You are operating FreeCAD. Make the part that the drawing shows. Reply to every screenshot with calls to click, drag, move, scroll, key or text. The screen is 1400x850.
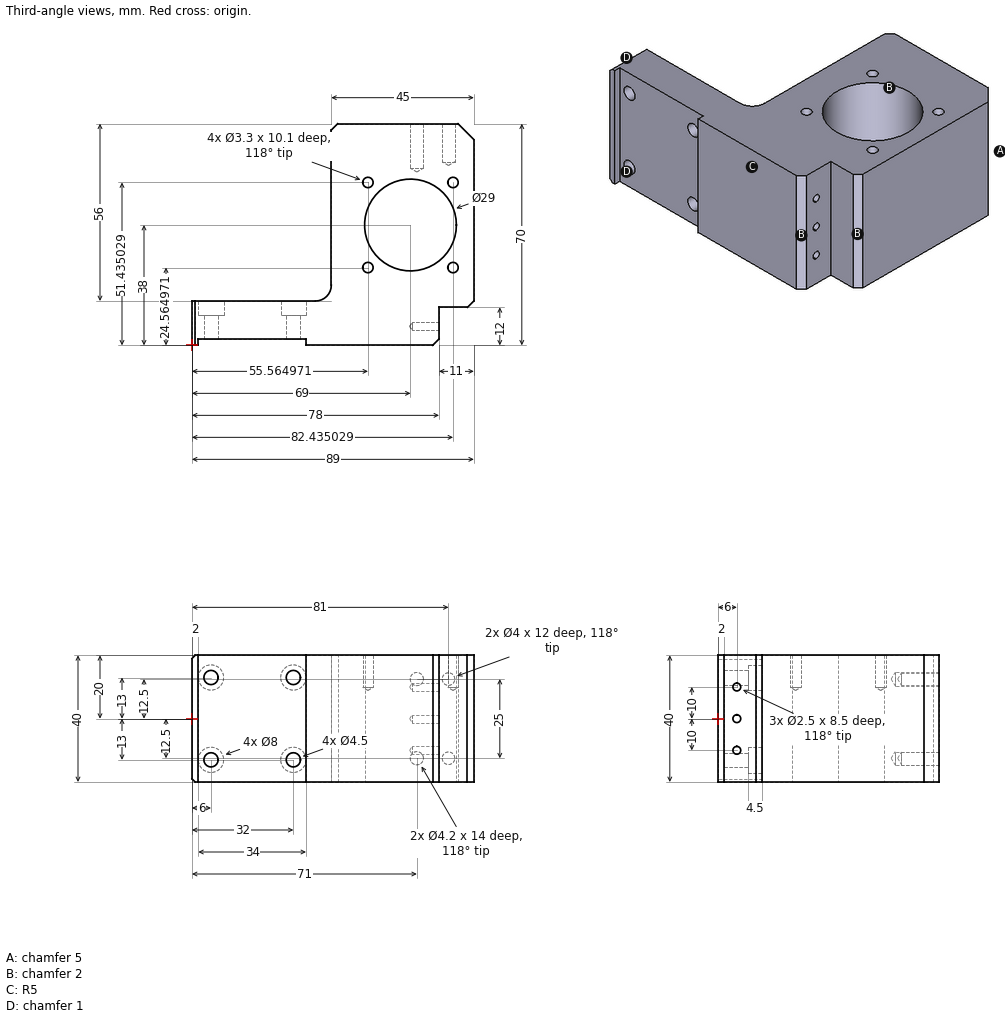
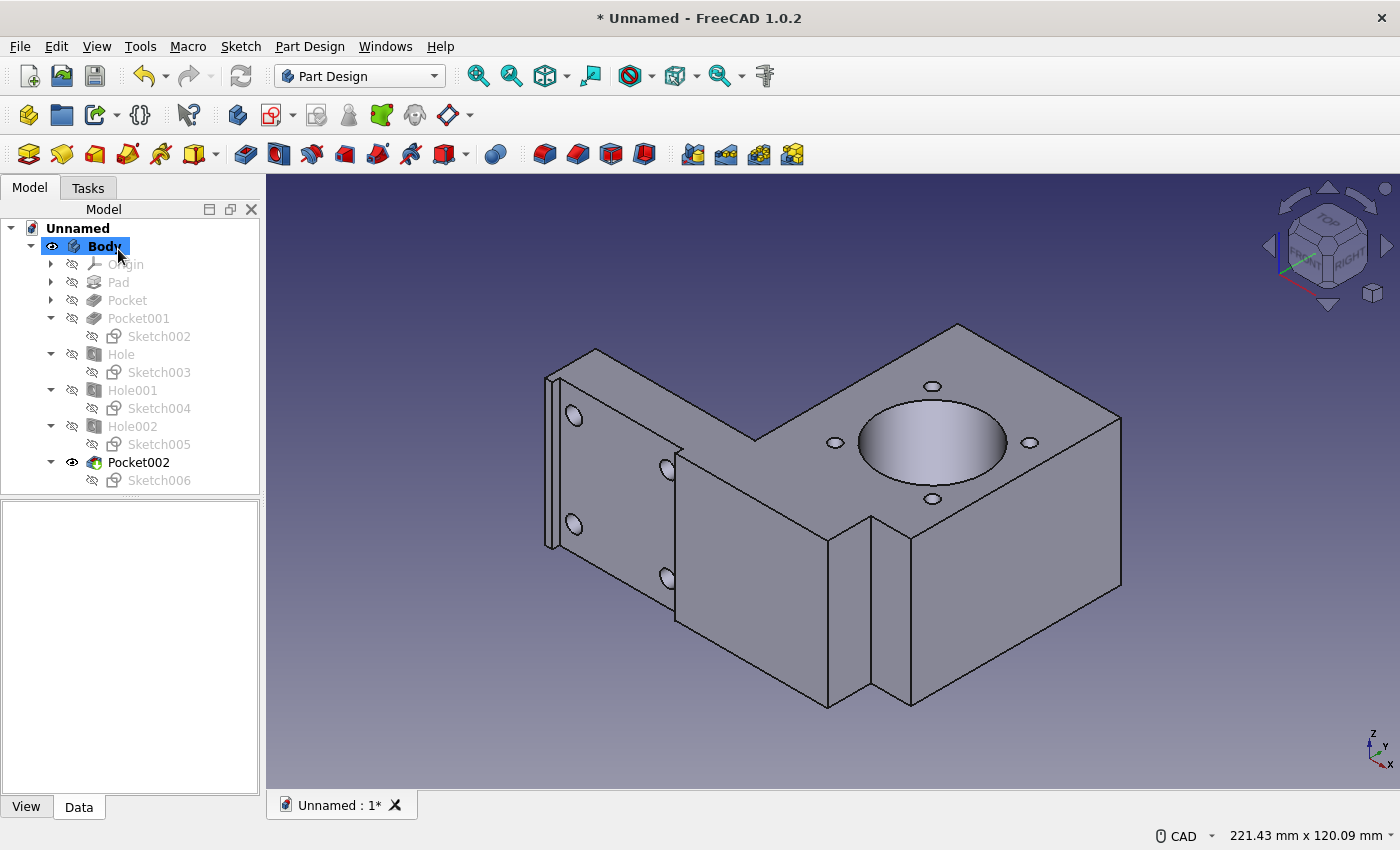
click(849, 563)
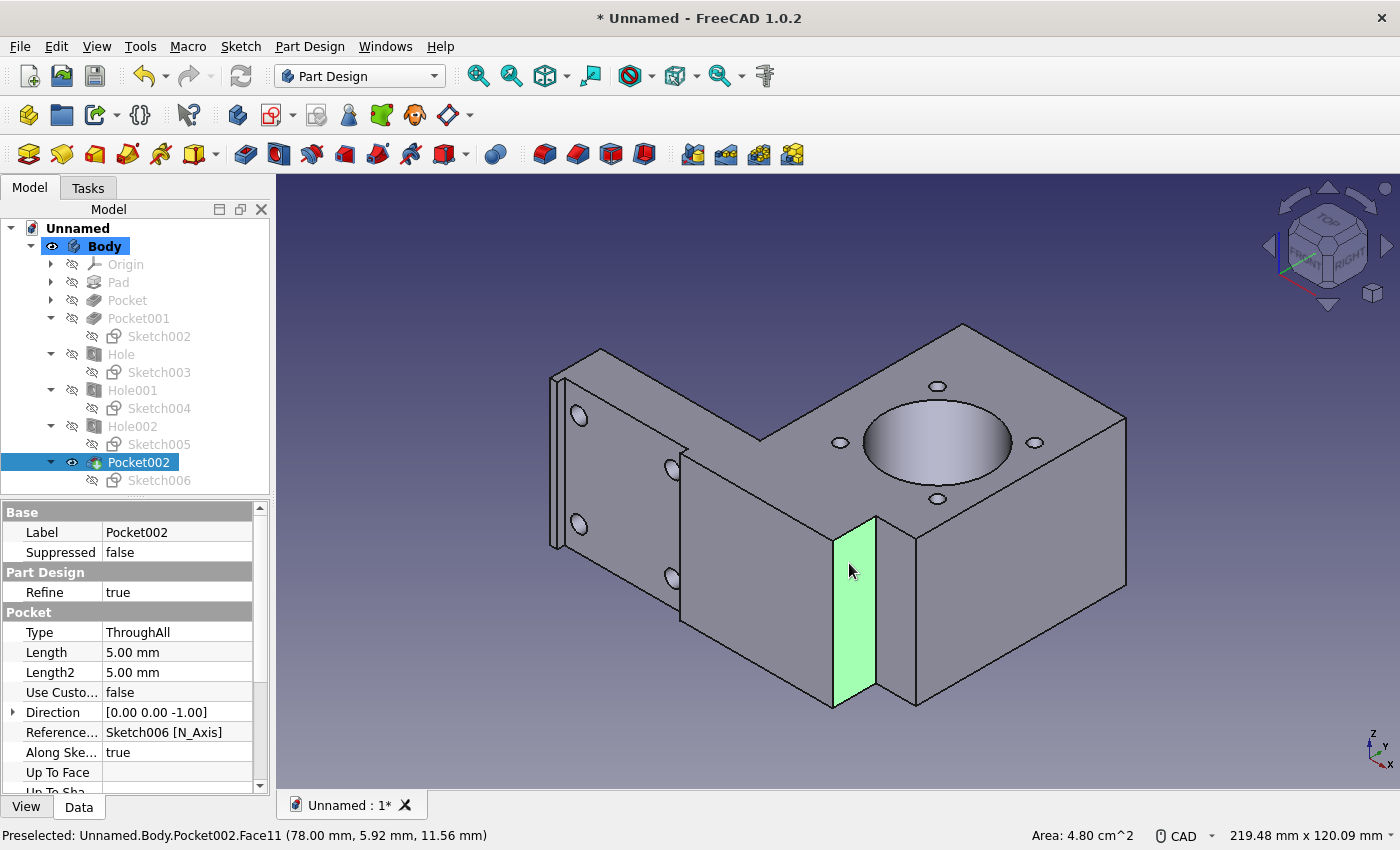
click(270, 116)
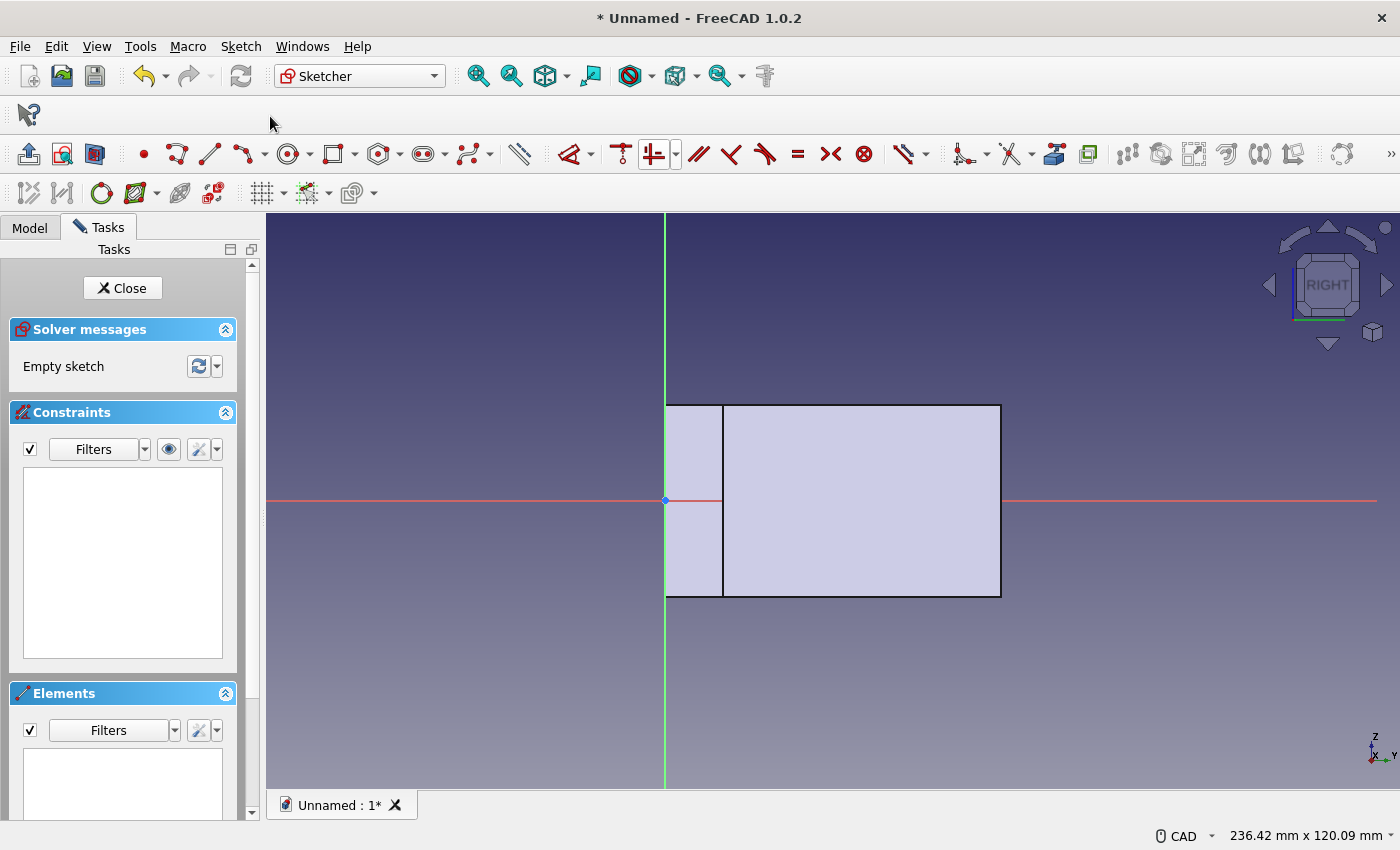
scroll(647, 501, up, 6)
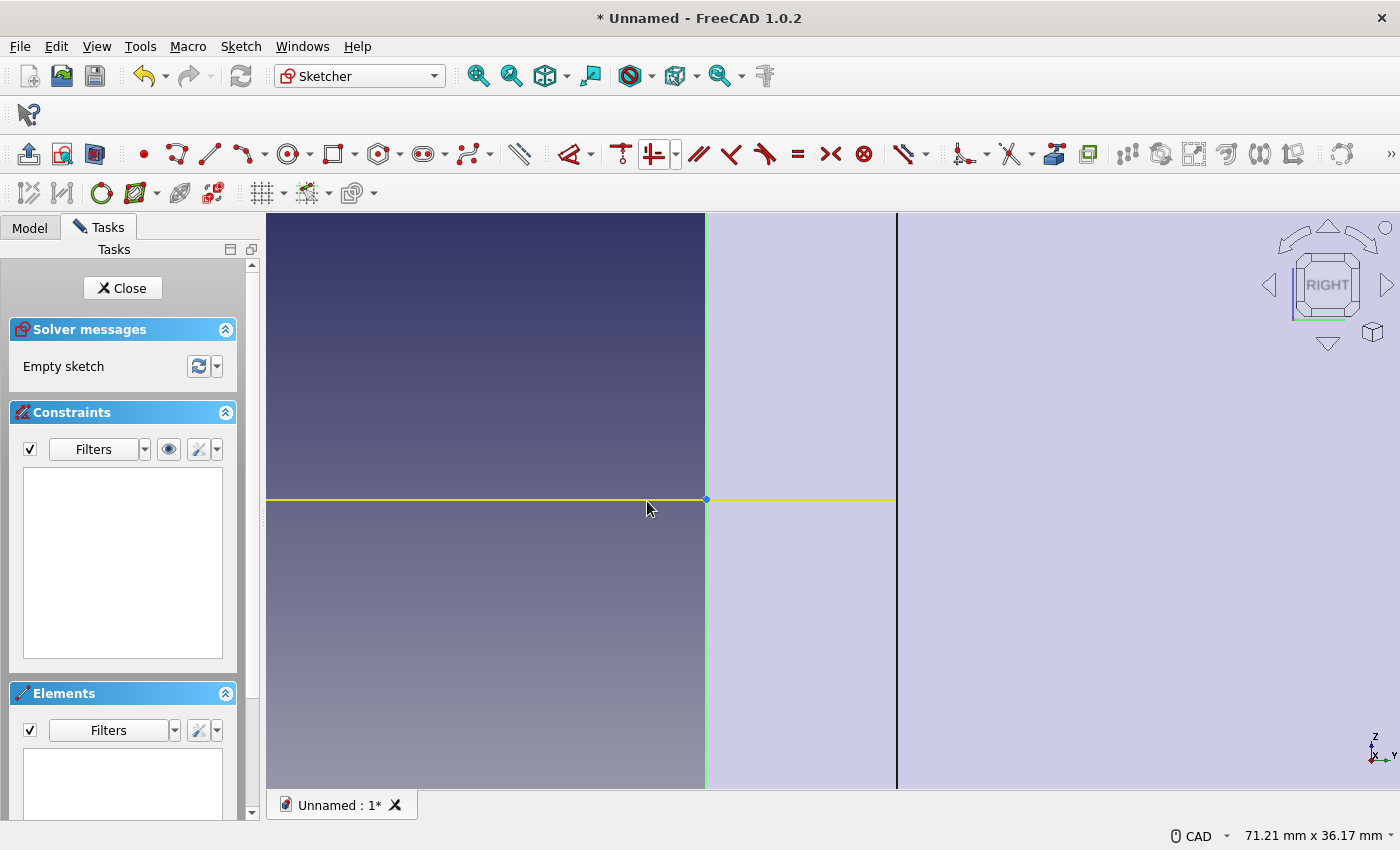
key(g)
key(c)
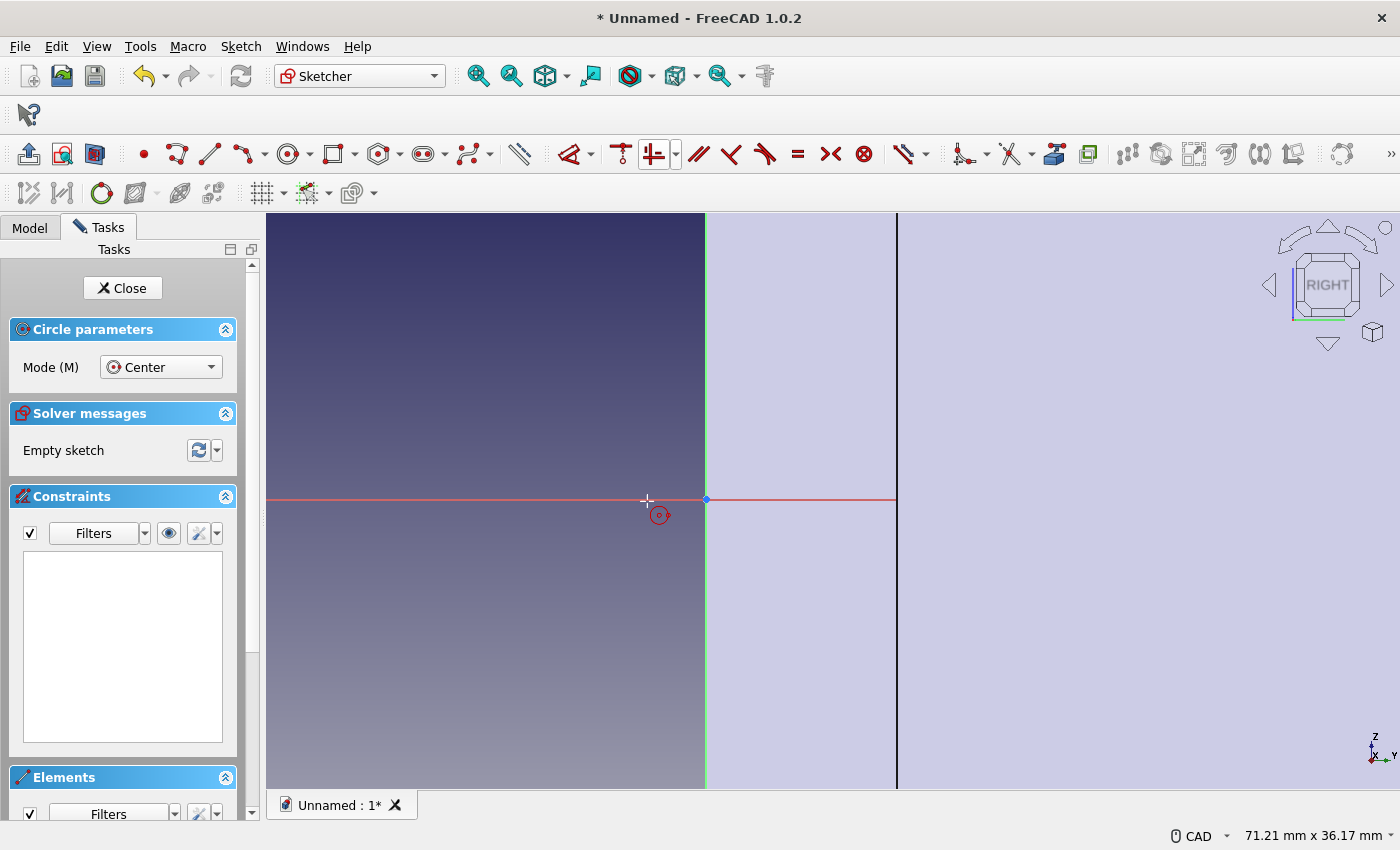
click(802, 341)
move(816, 327)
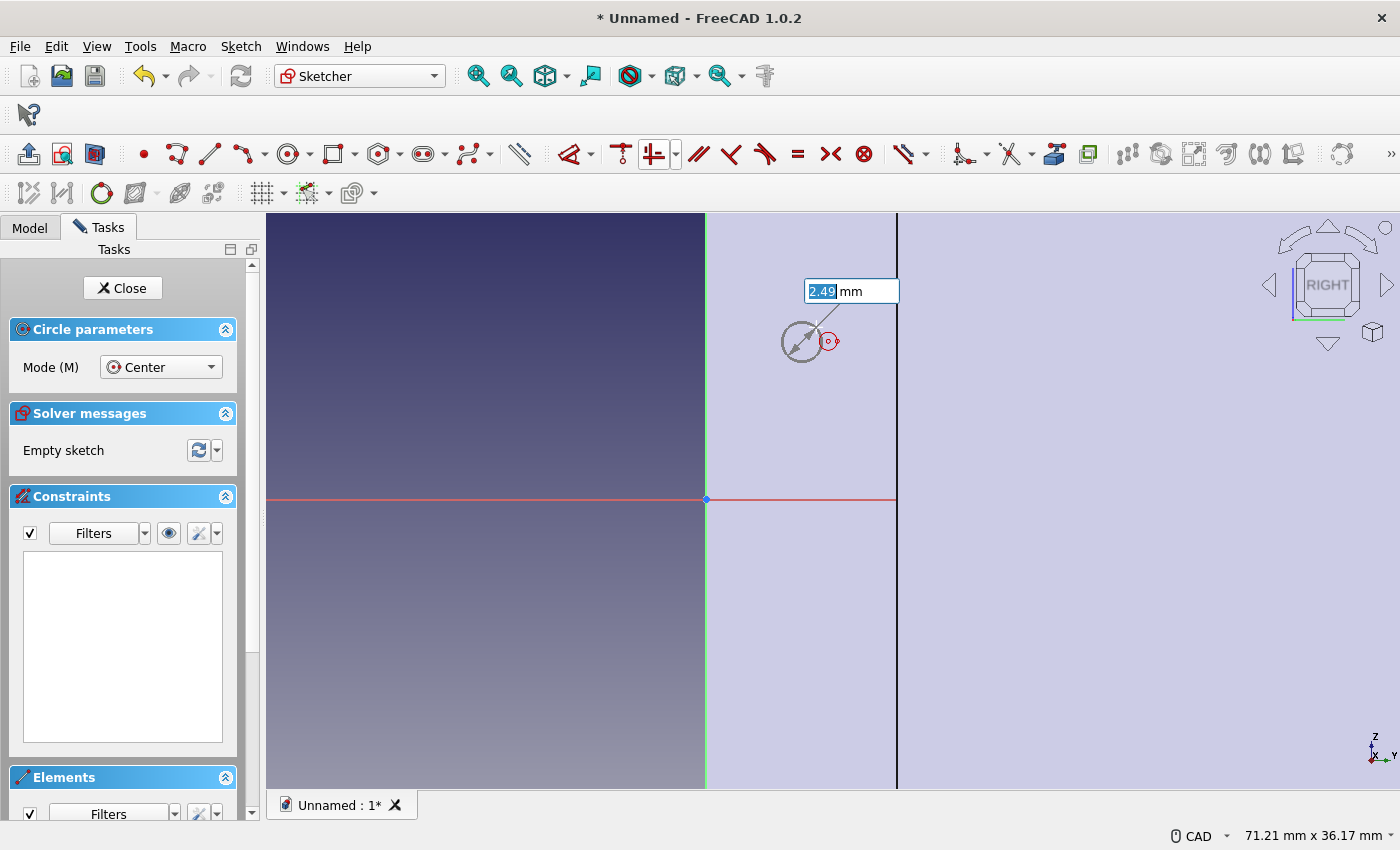
text(2.5)
key(Return)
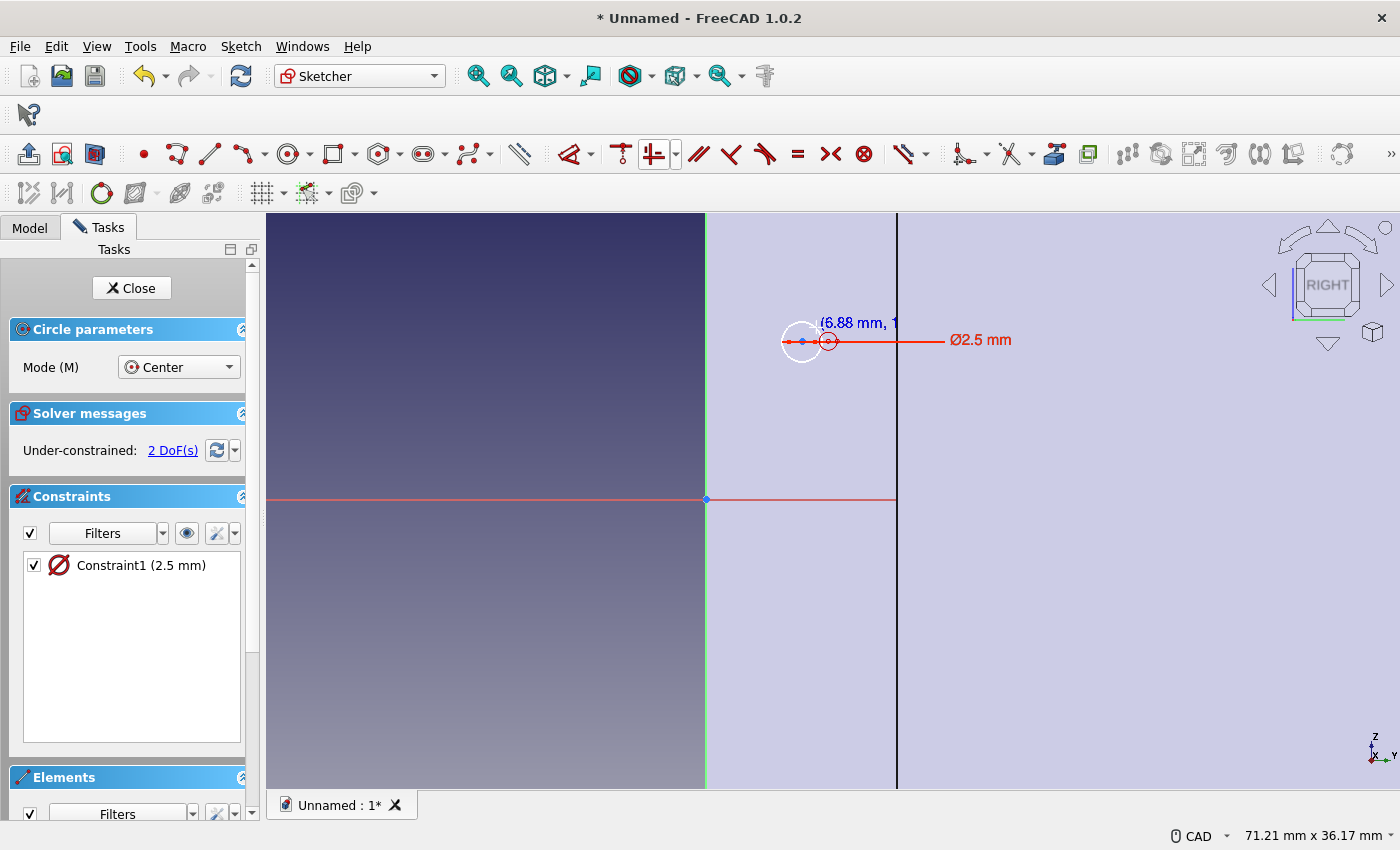
click(802, 500)
move(816, 486)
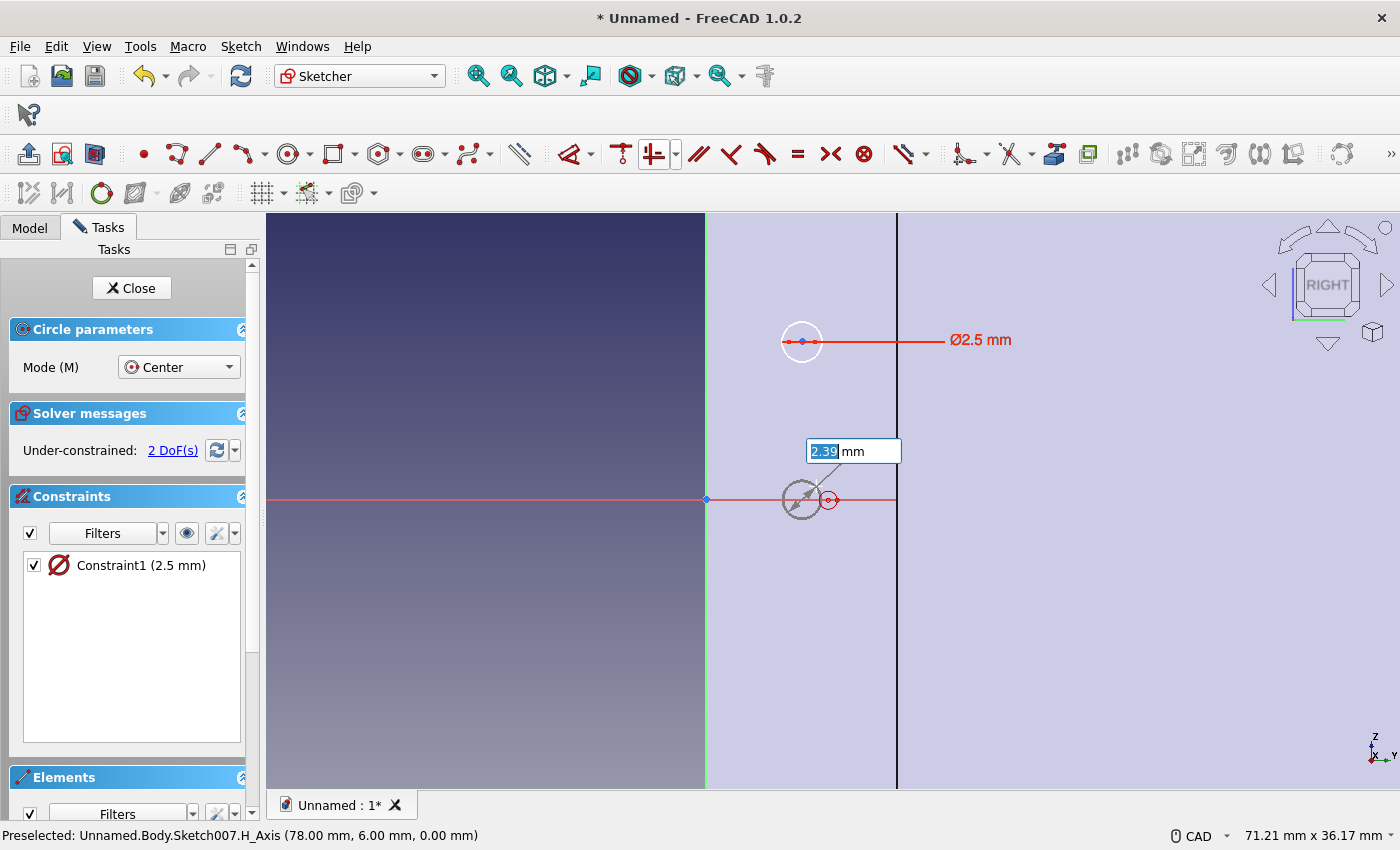
text(2.5)
key(Return)